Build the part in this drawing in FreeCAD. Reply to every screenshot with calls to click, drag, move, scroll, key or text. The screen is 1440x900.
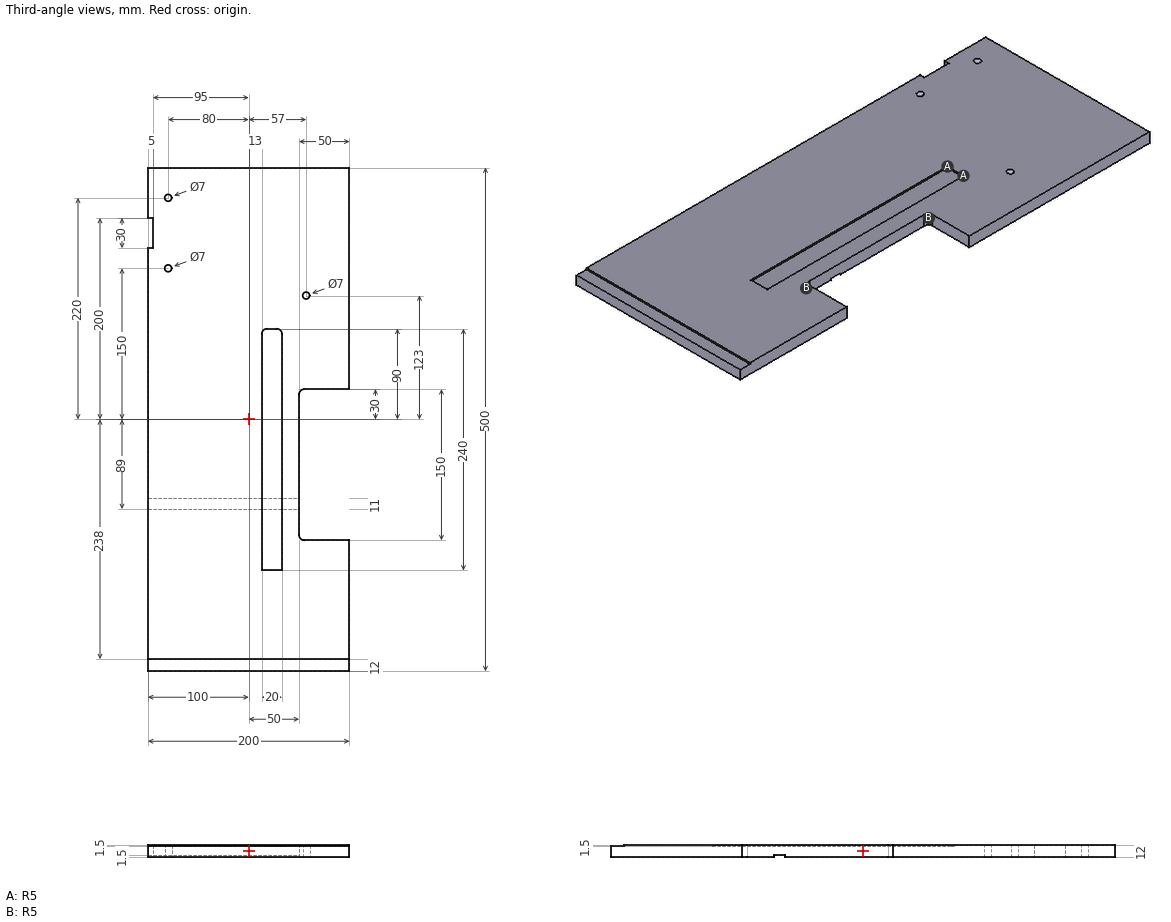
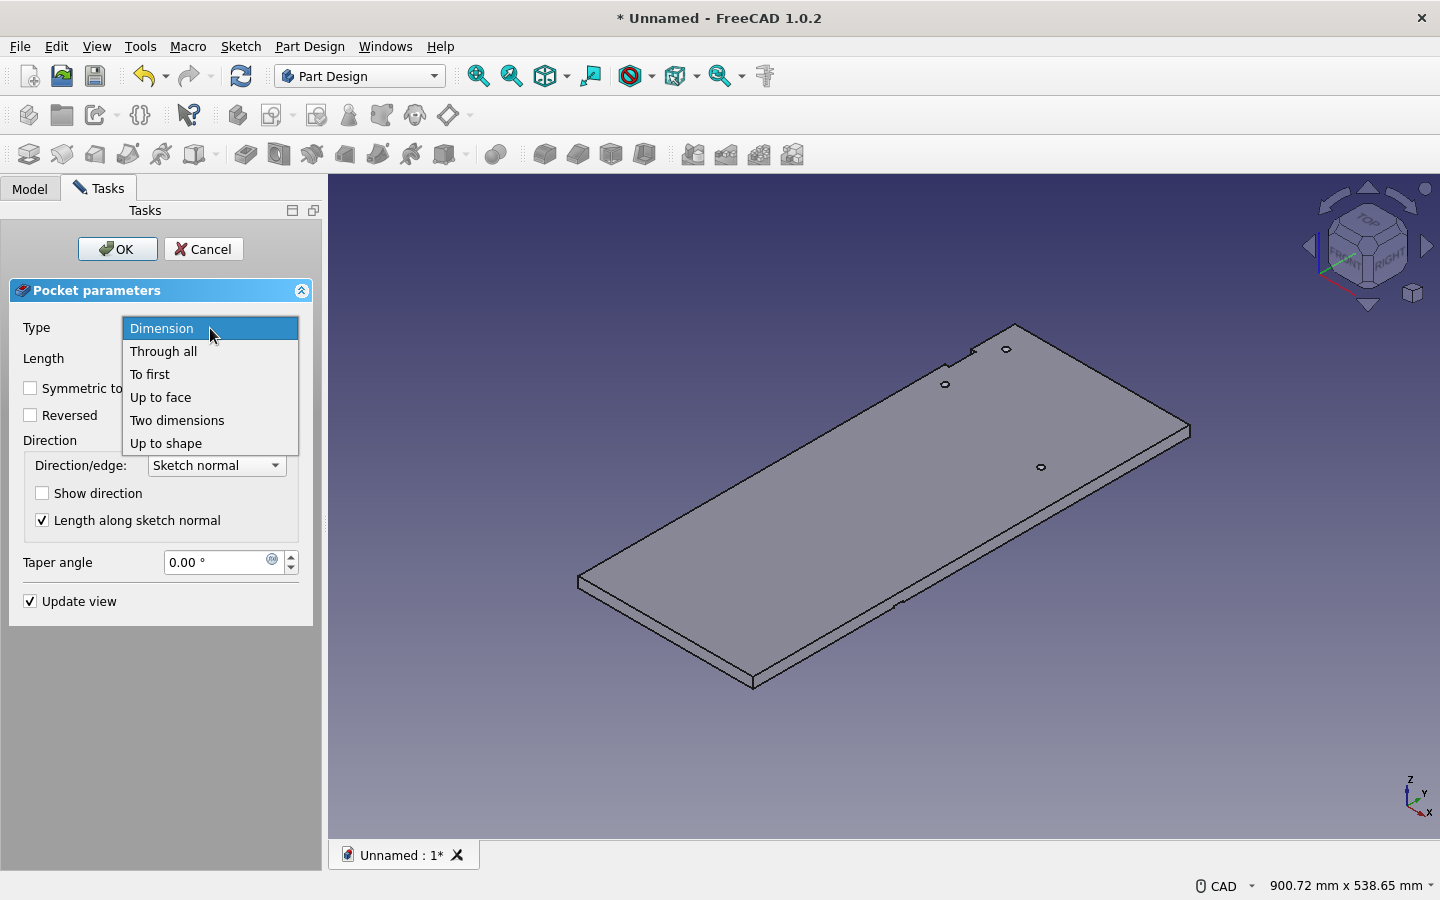
click(208, 374)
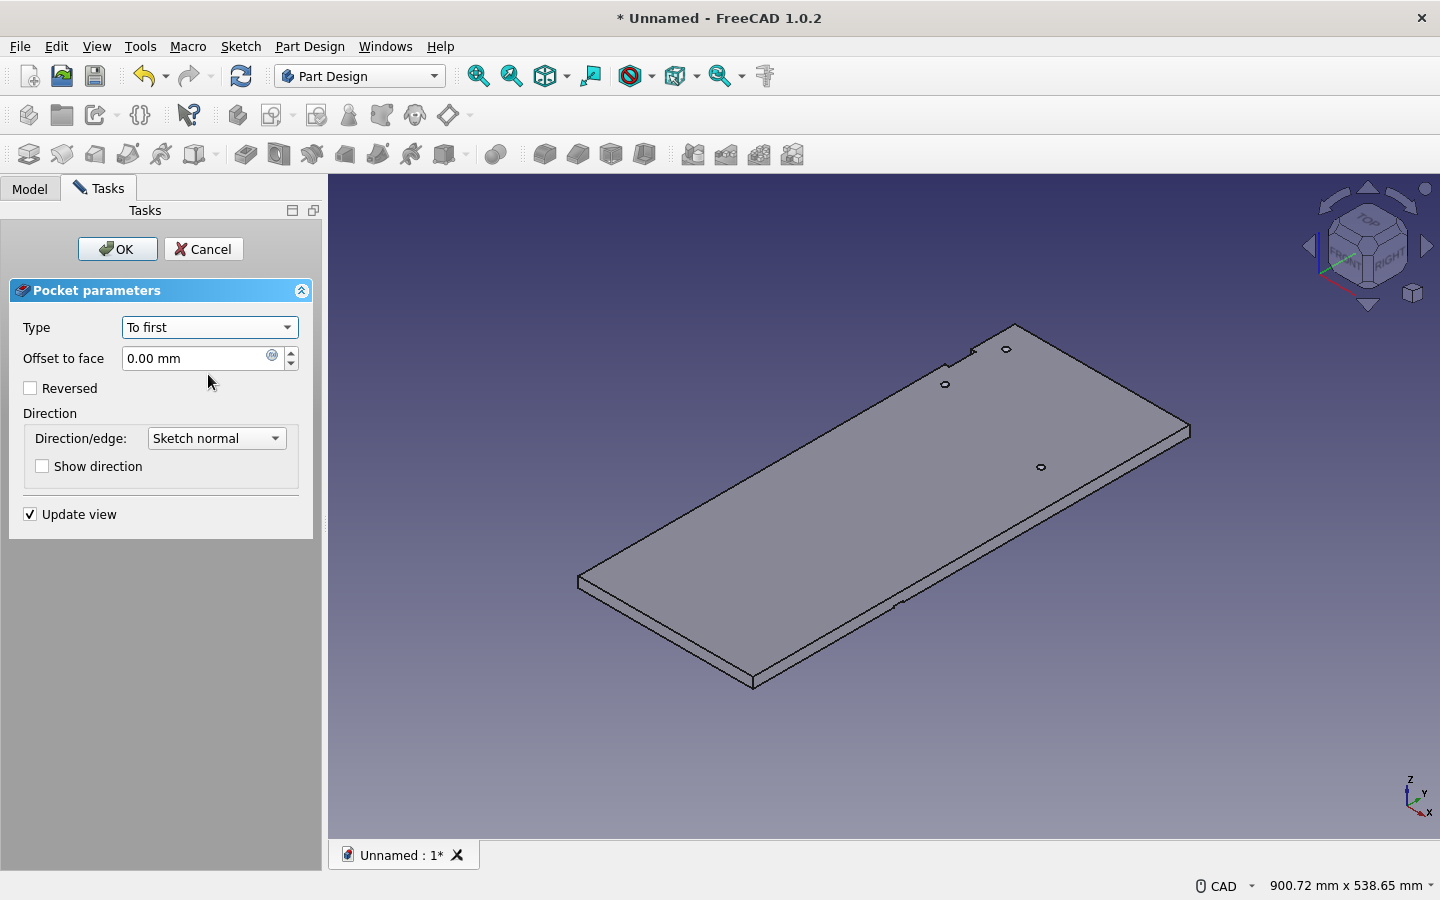
click(118, 249)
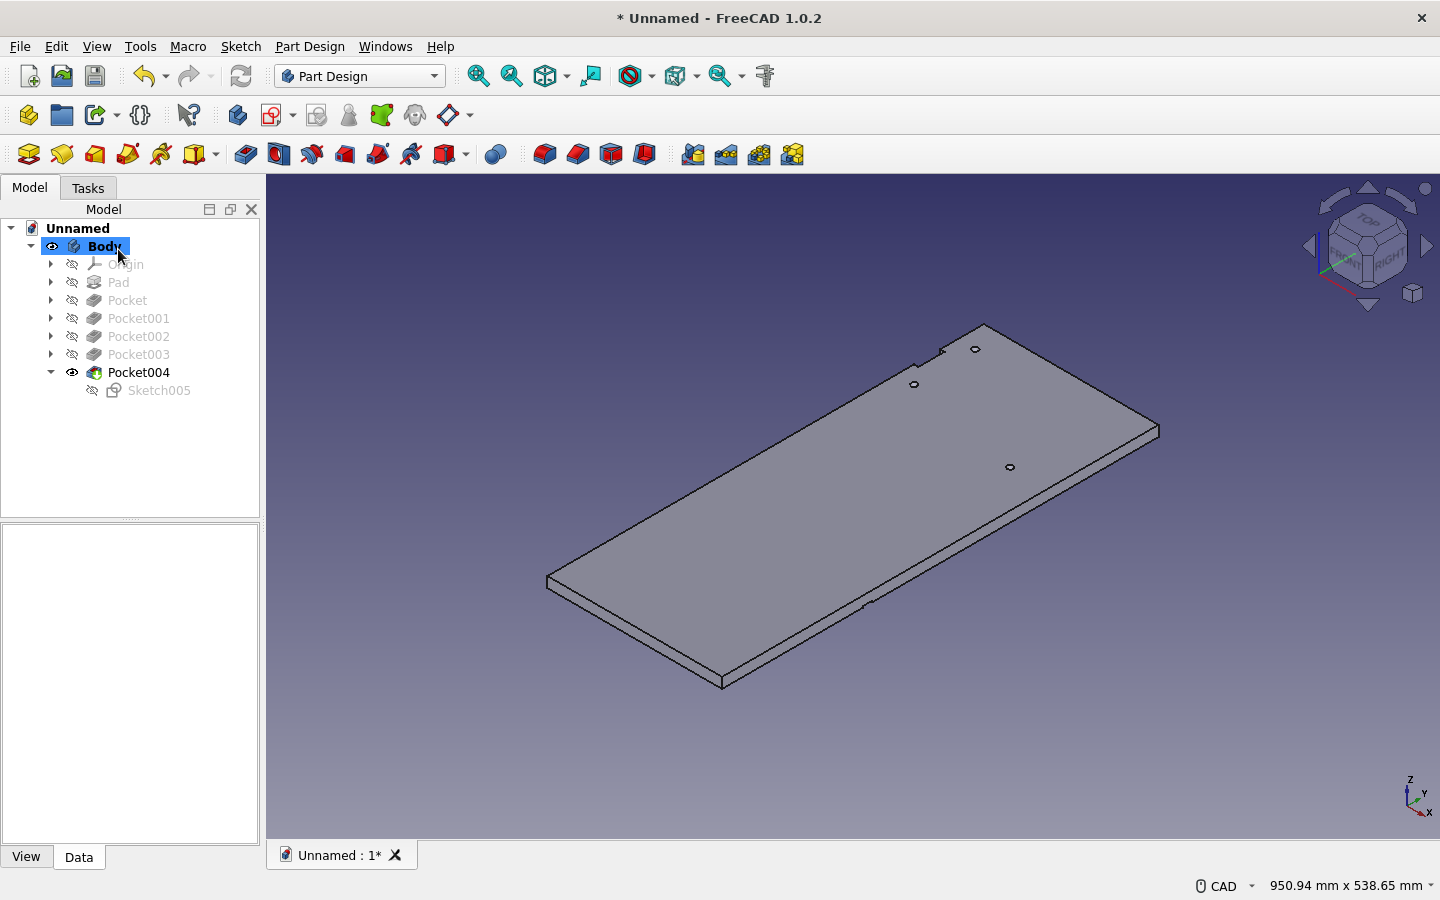
click(853, 499)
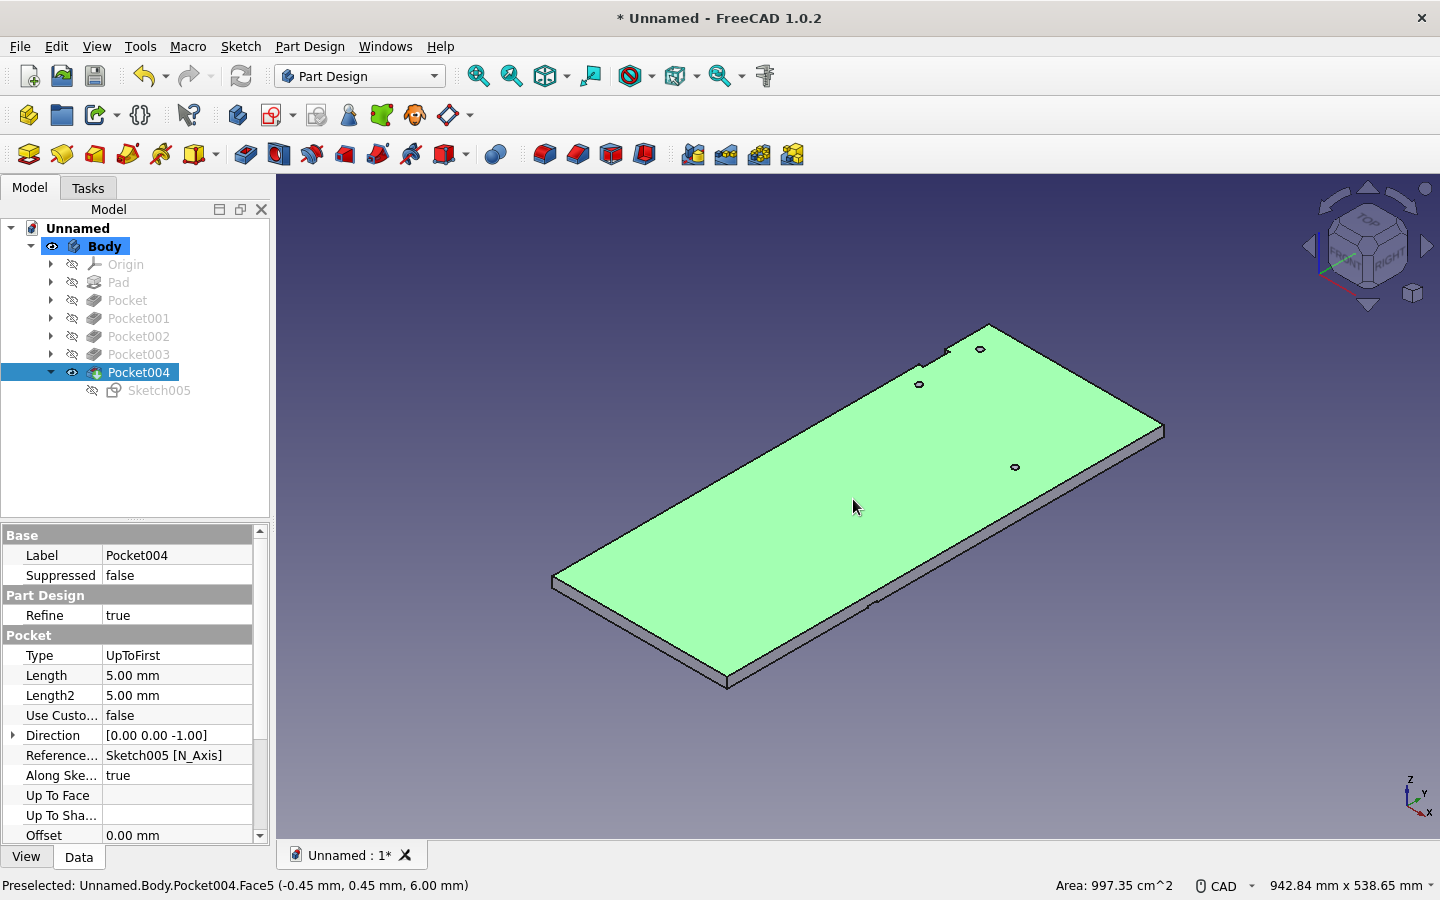
click(270, 116)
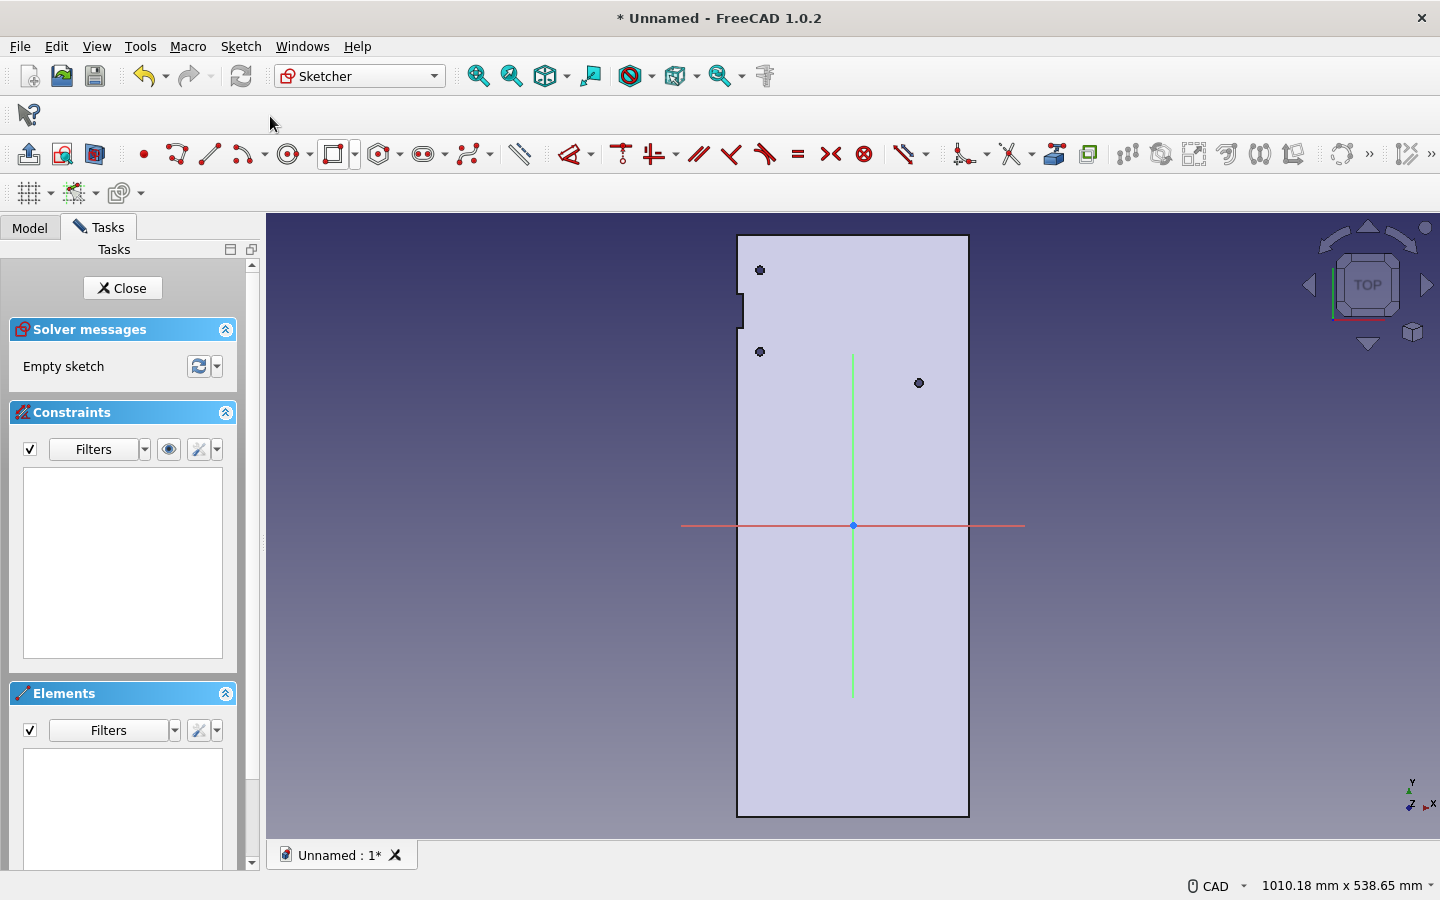
scroll(1050, 632, up, 2)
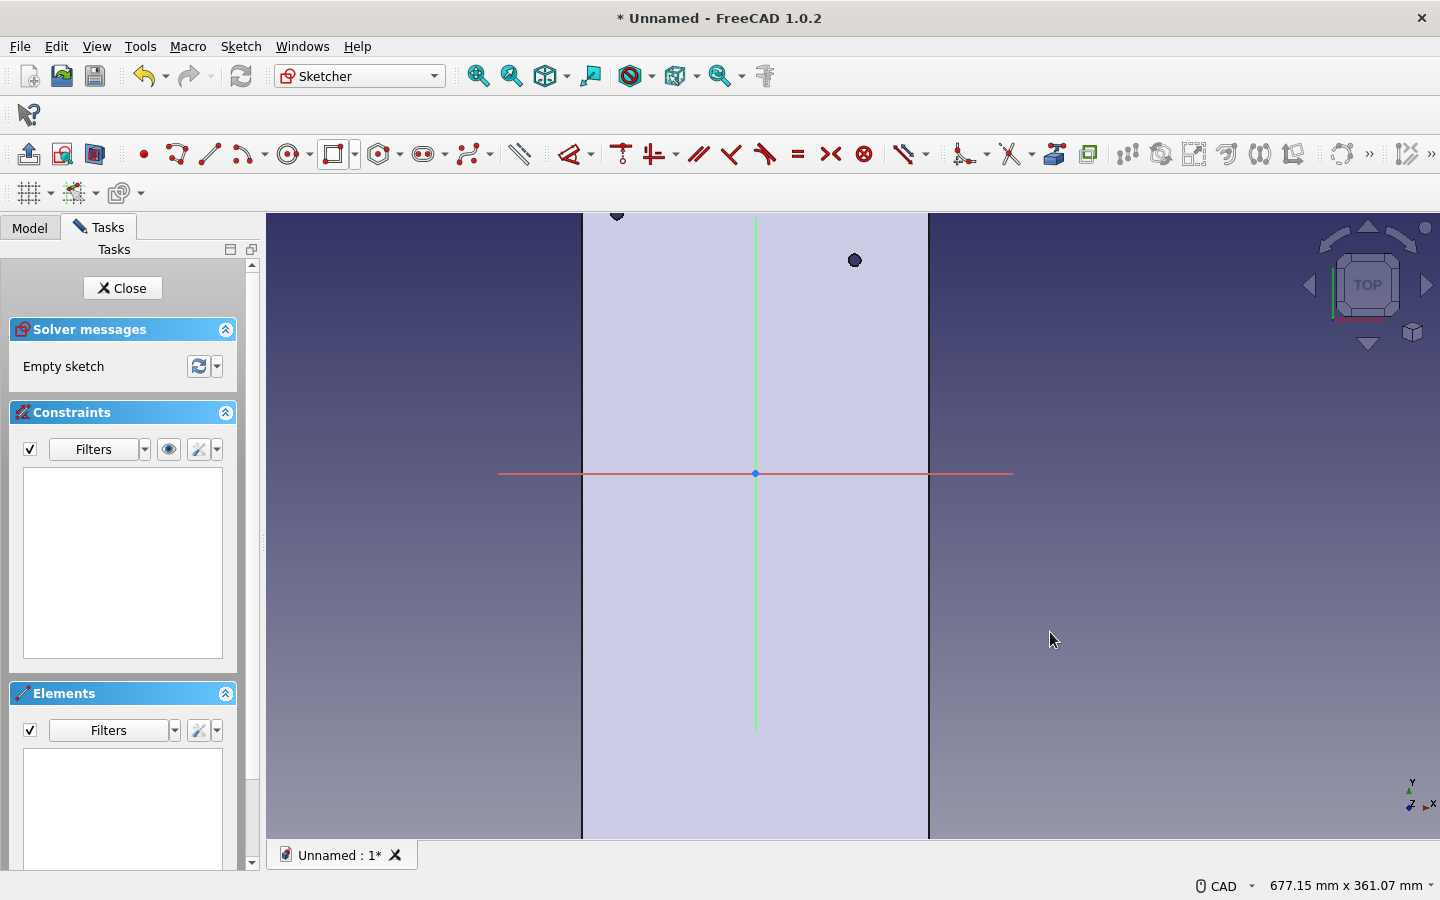
click(332, 154)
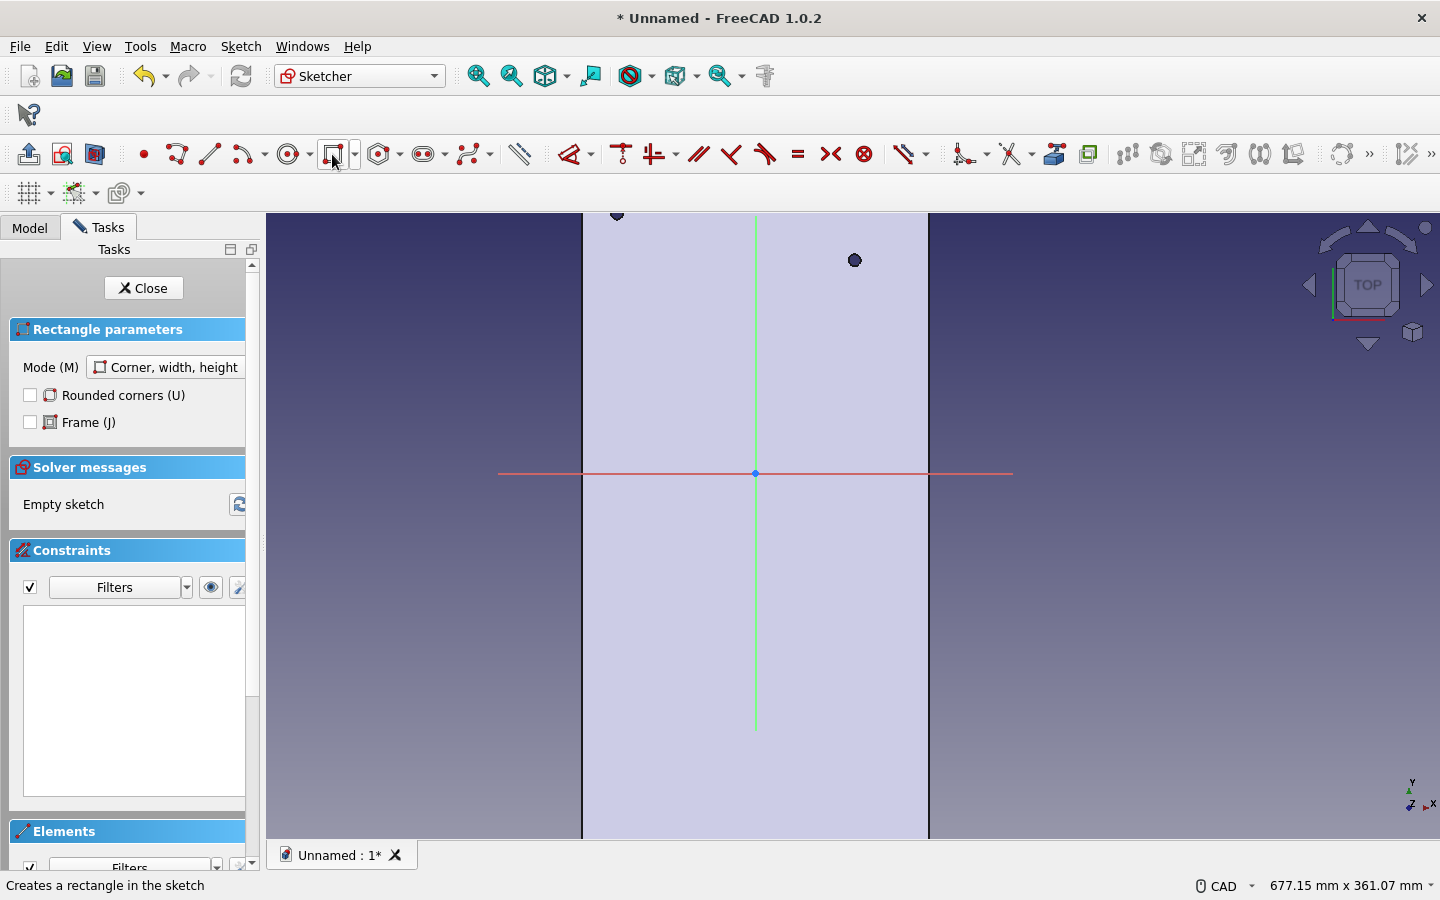
click(778, 317)
move(813, 734)